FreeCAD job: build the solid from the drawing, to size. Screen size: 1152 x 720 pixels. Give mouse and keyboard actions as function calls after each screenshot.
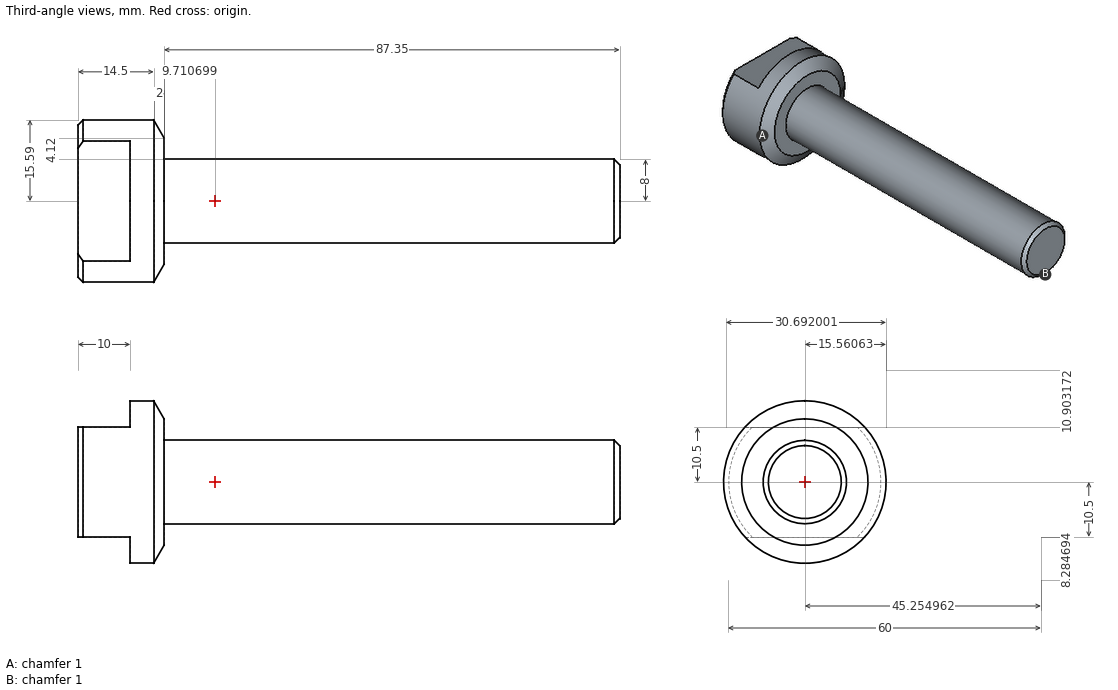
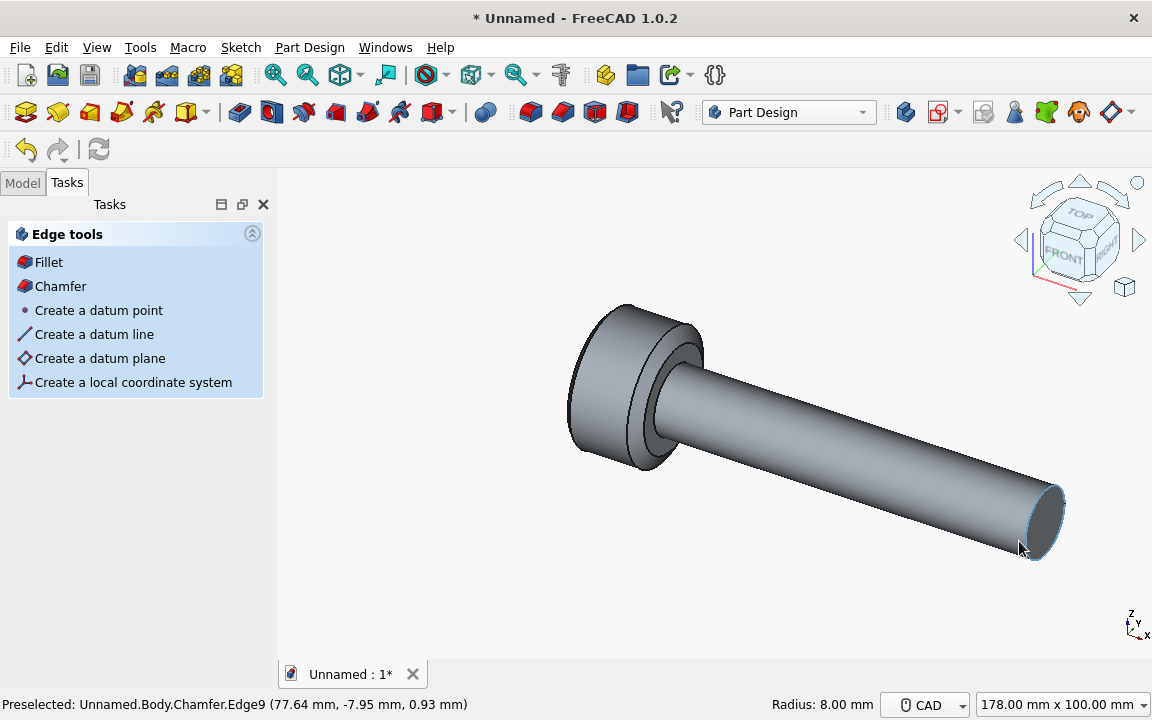
click(564, 112)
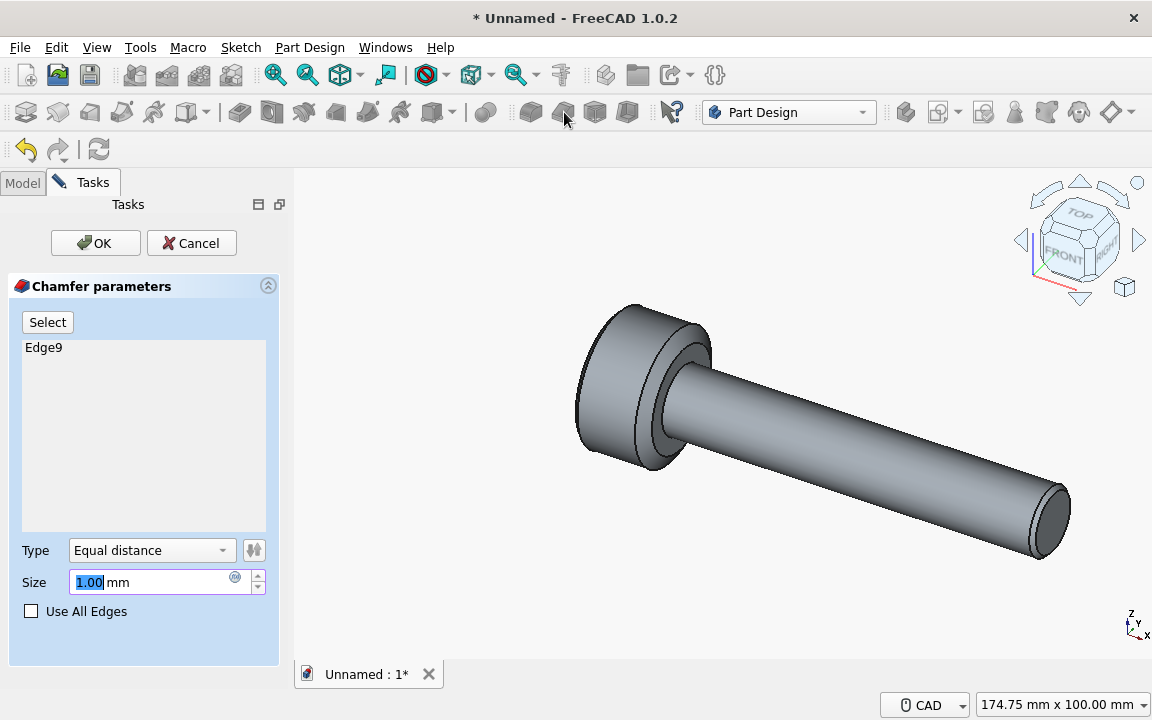
text(1)
key(Tab)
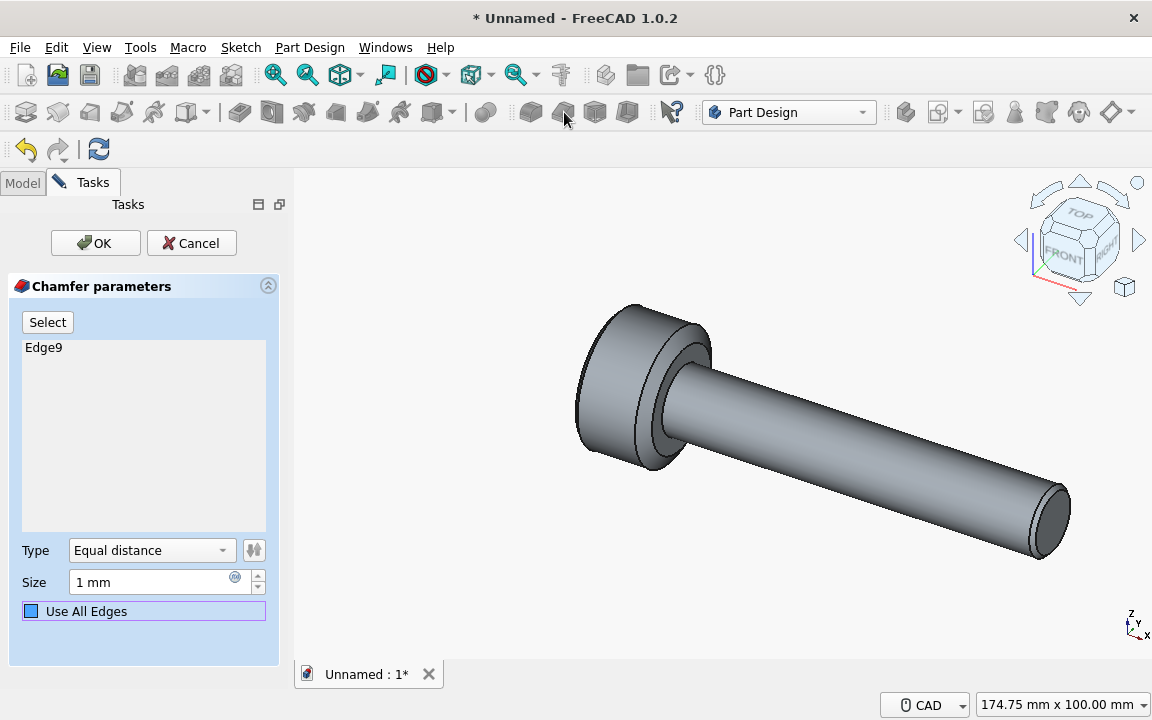
click(96, 243)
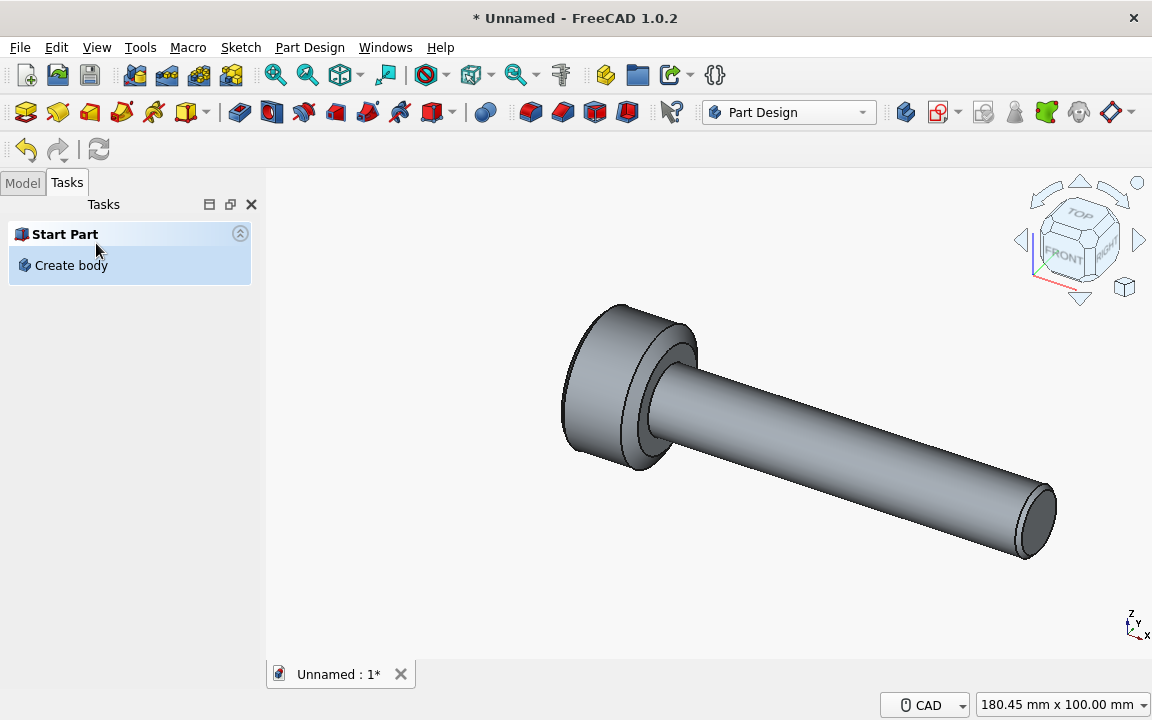
key(6)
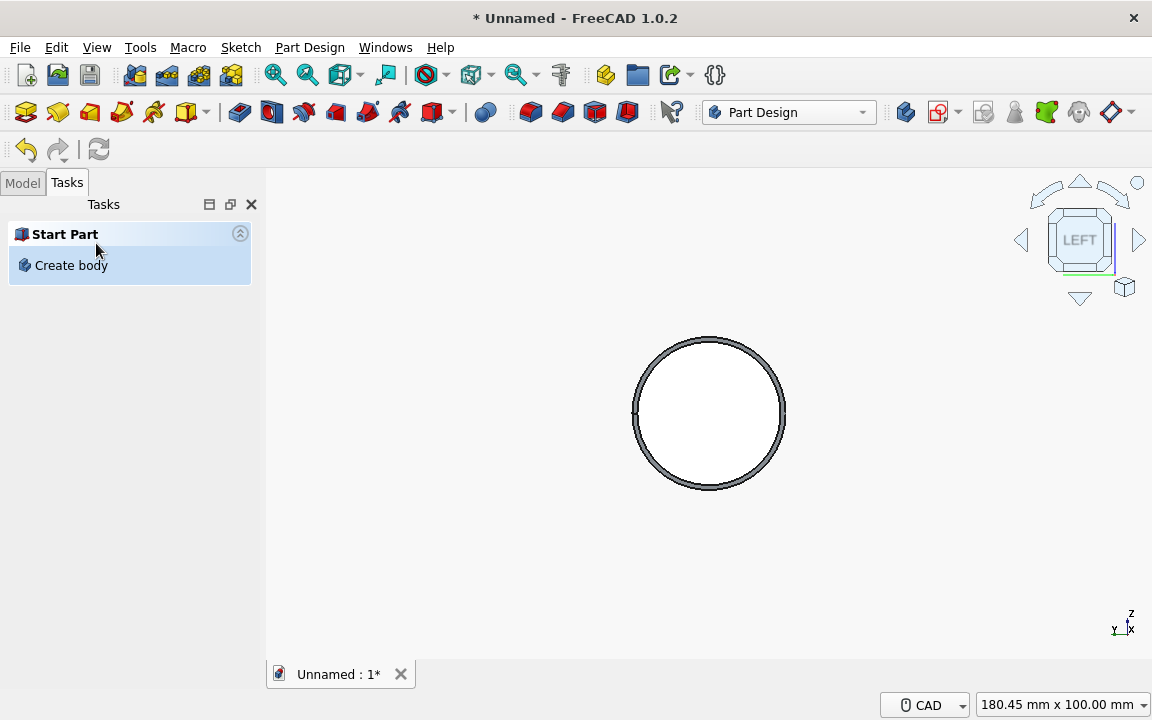
key(v)
key(f)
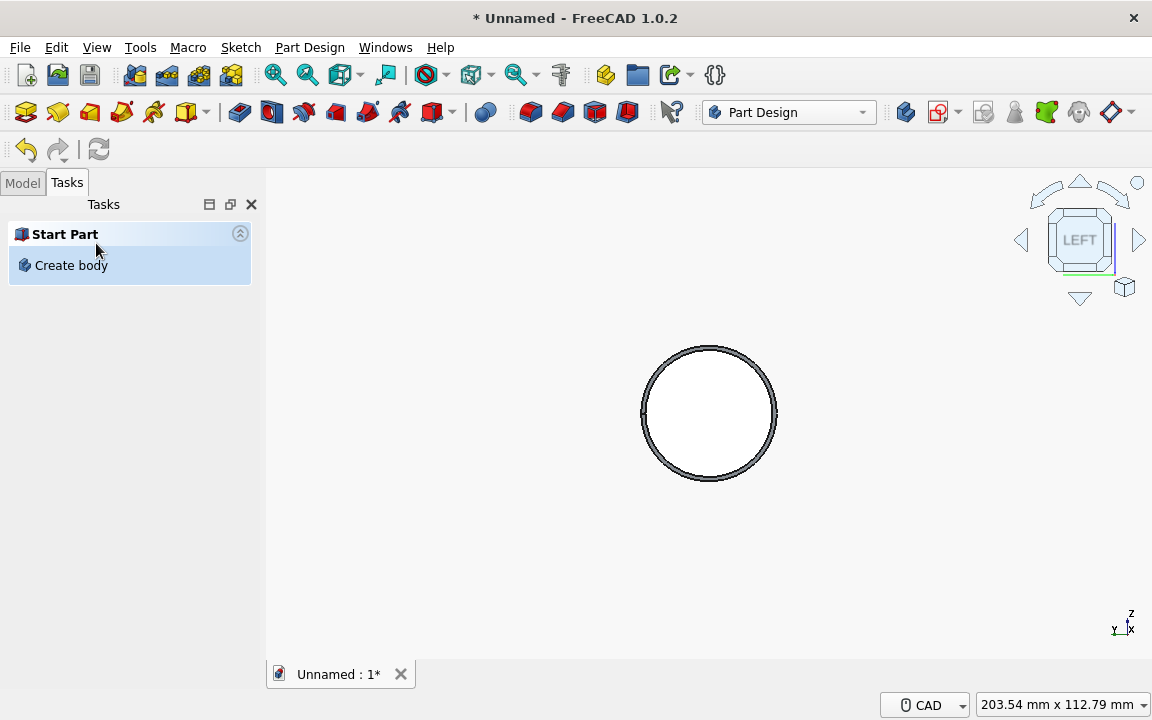
click(709, 412)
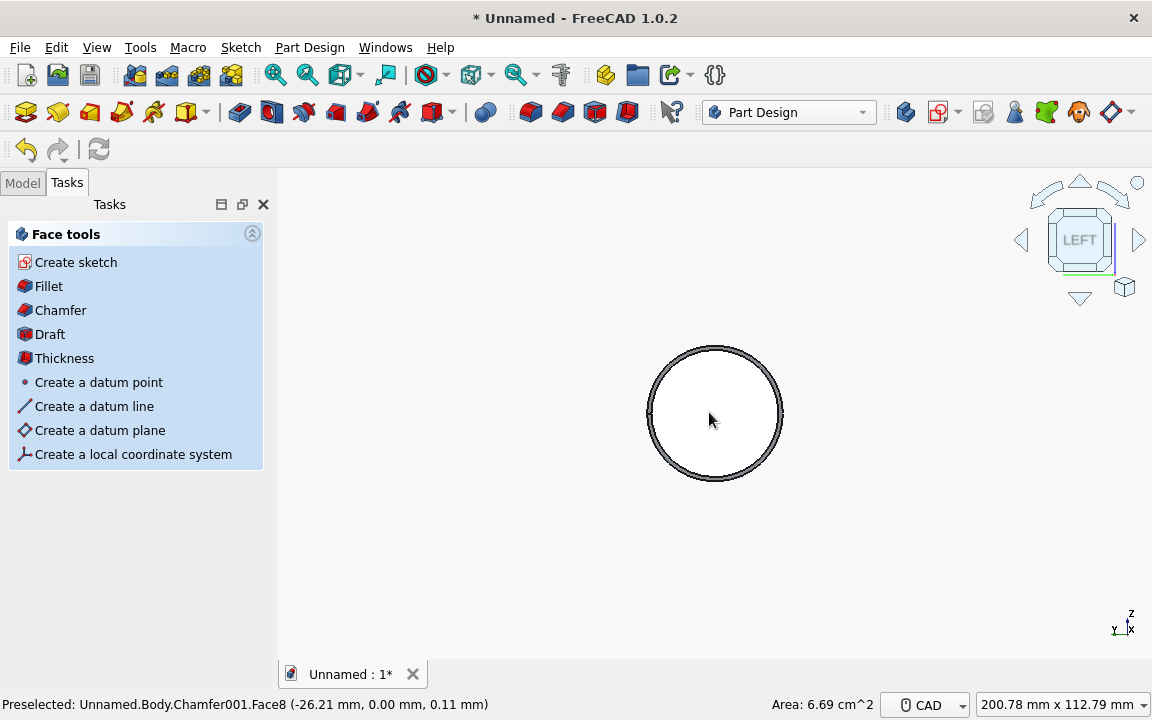
click(938, 112)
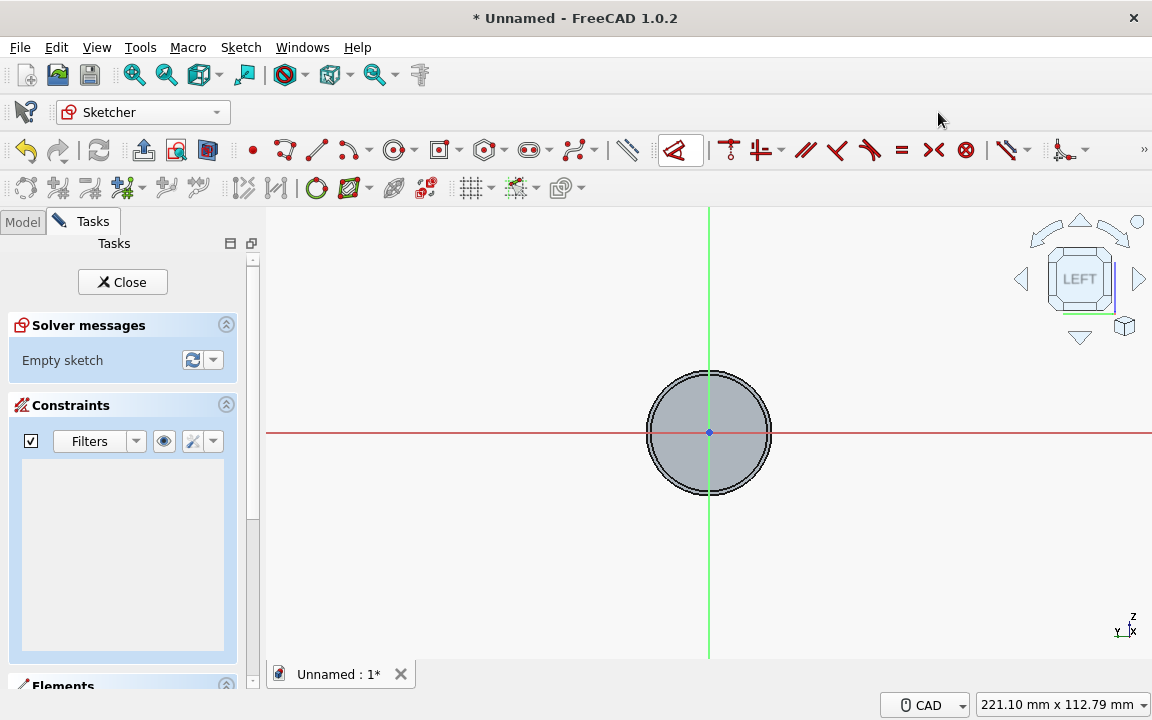
scroll(659, 421, up, 3)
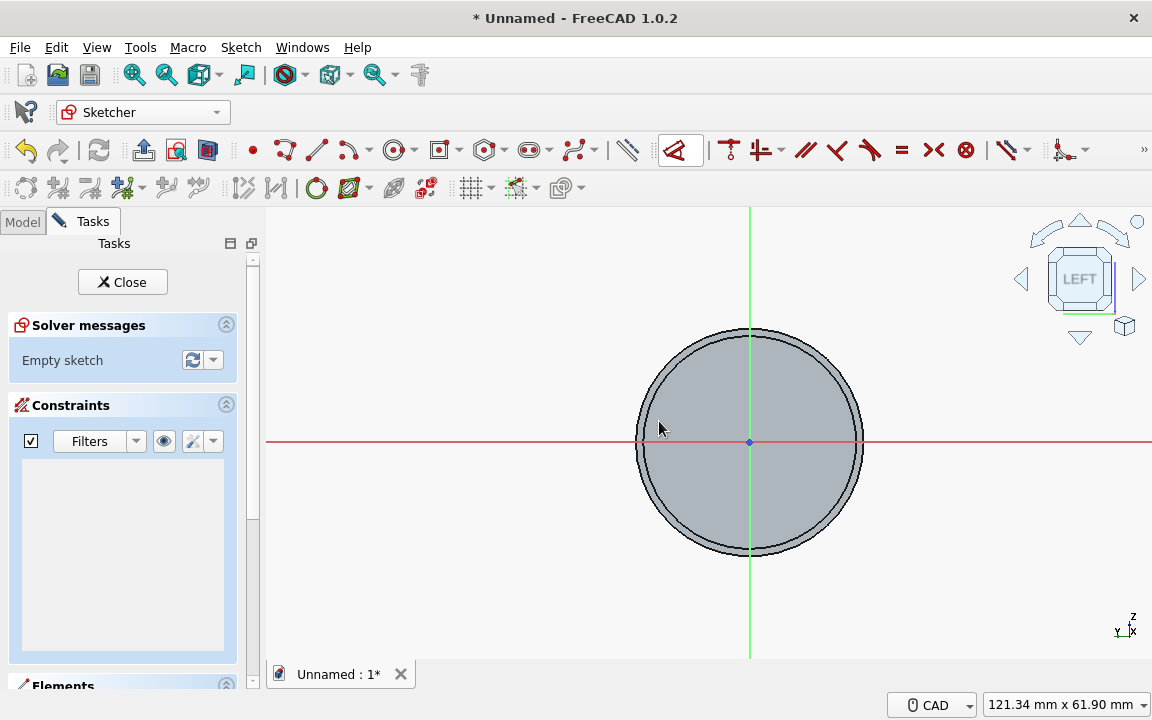
click(462, 150)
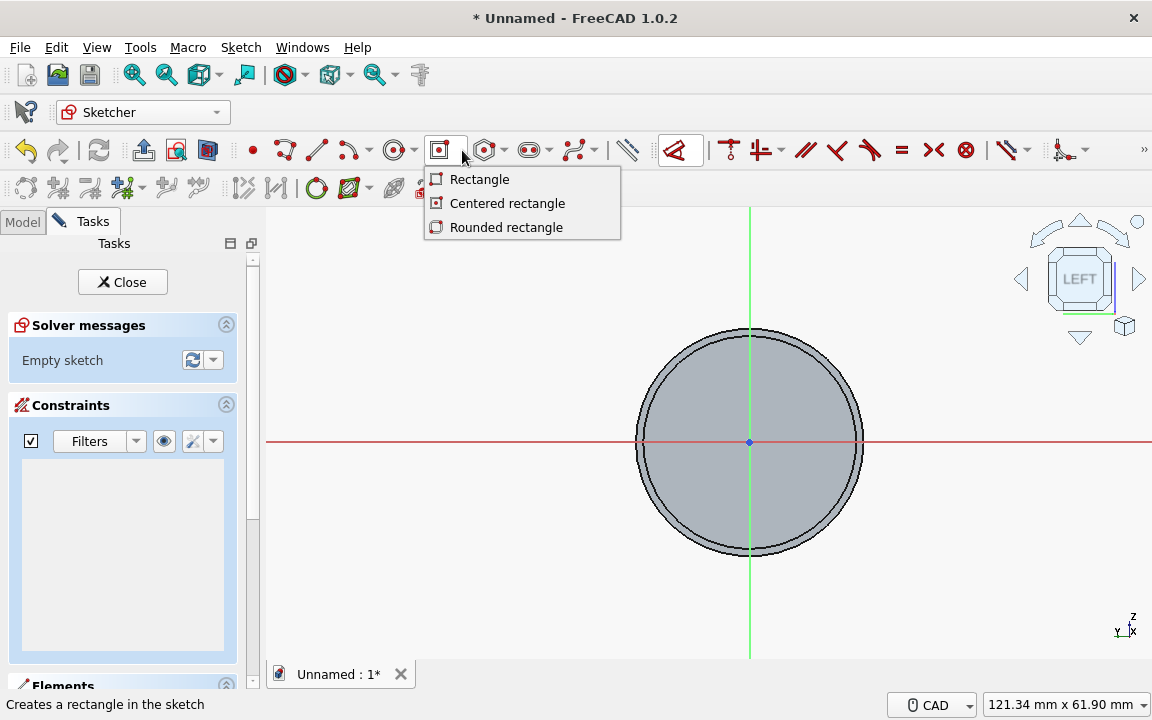
click(522, 179)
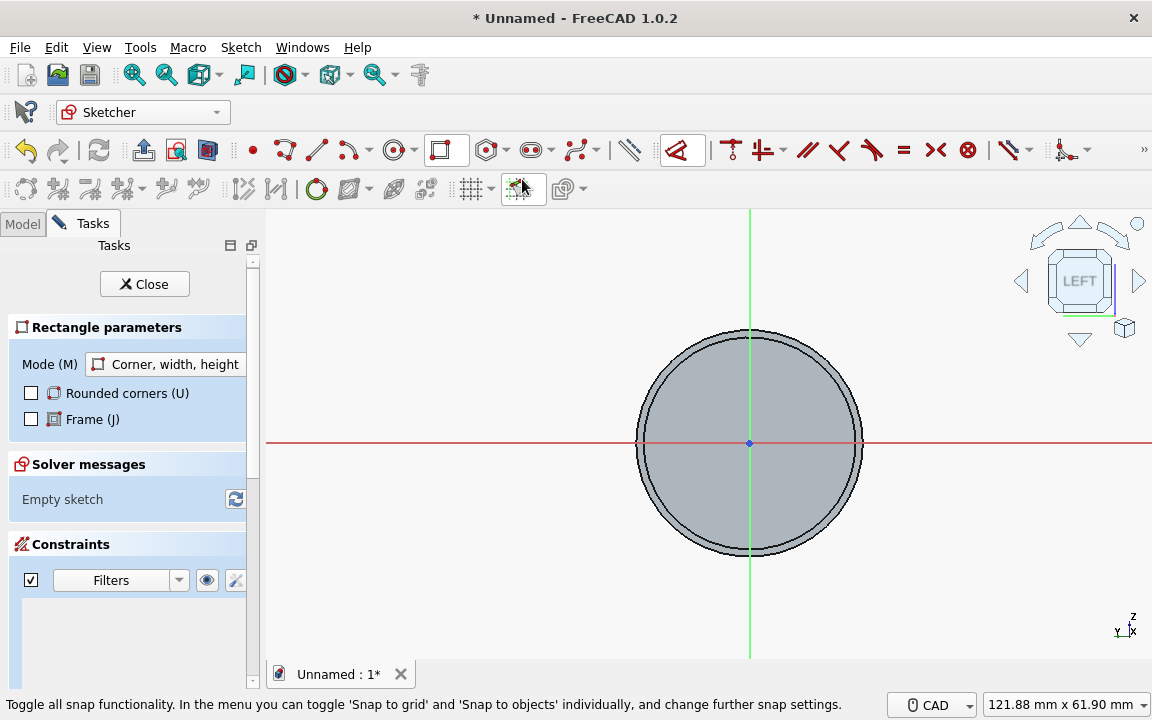
click(421, 520)
click(857, 580)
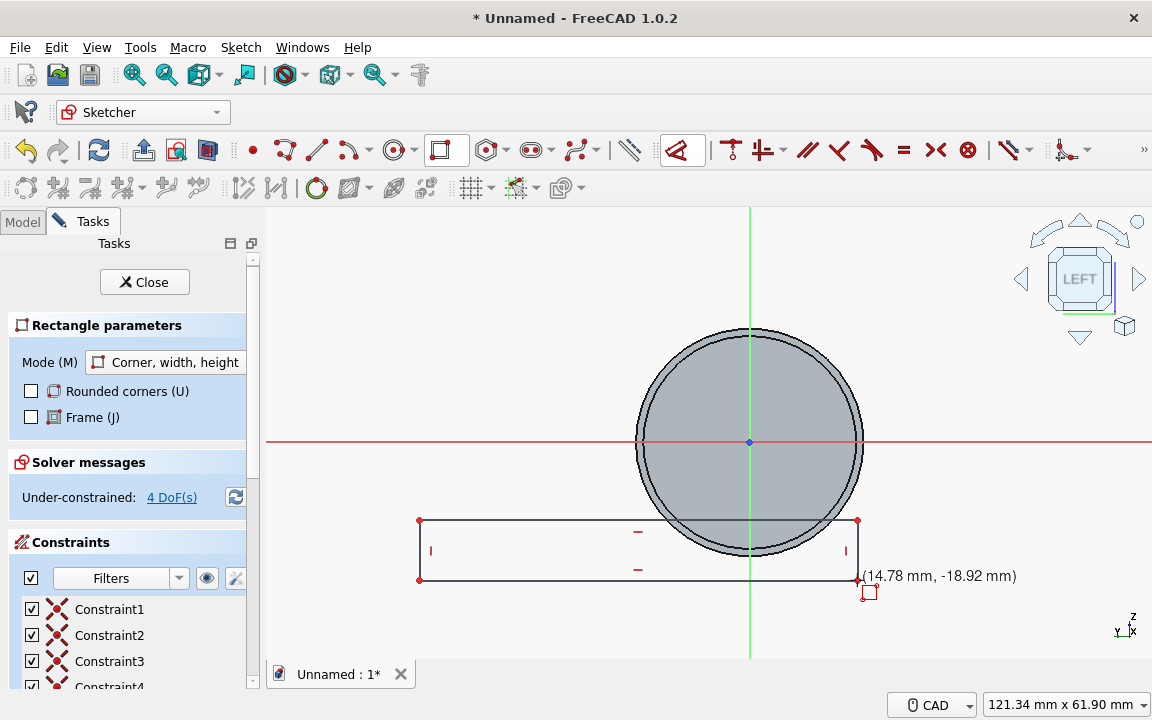
click(636, 286)
click(860, 366)
key(Escape)